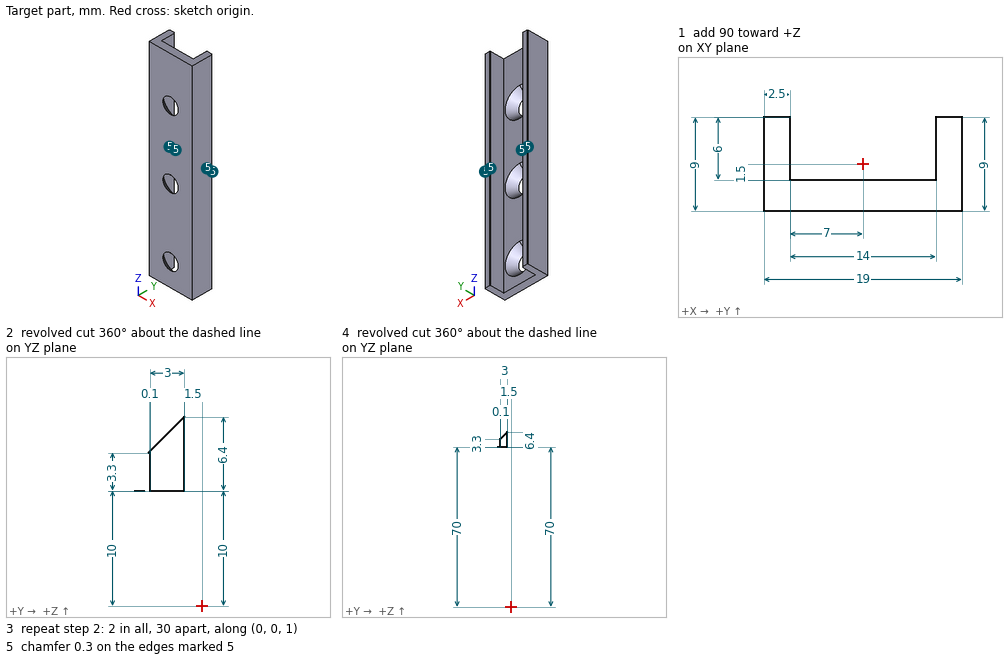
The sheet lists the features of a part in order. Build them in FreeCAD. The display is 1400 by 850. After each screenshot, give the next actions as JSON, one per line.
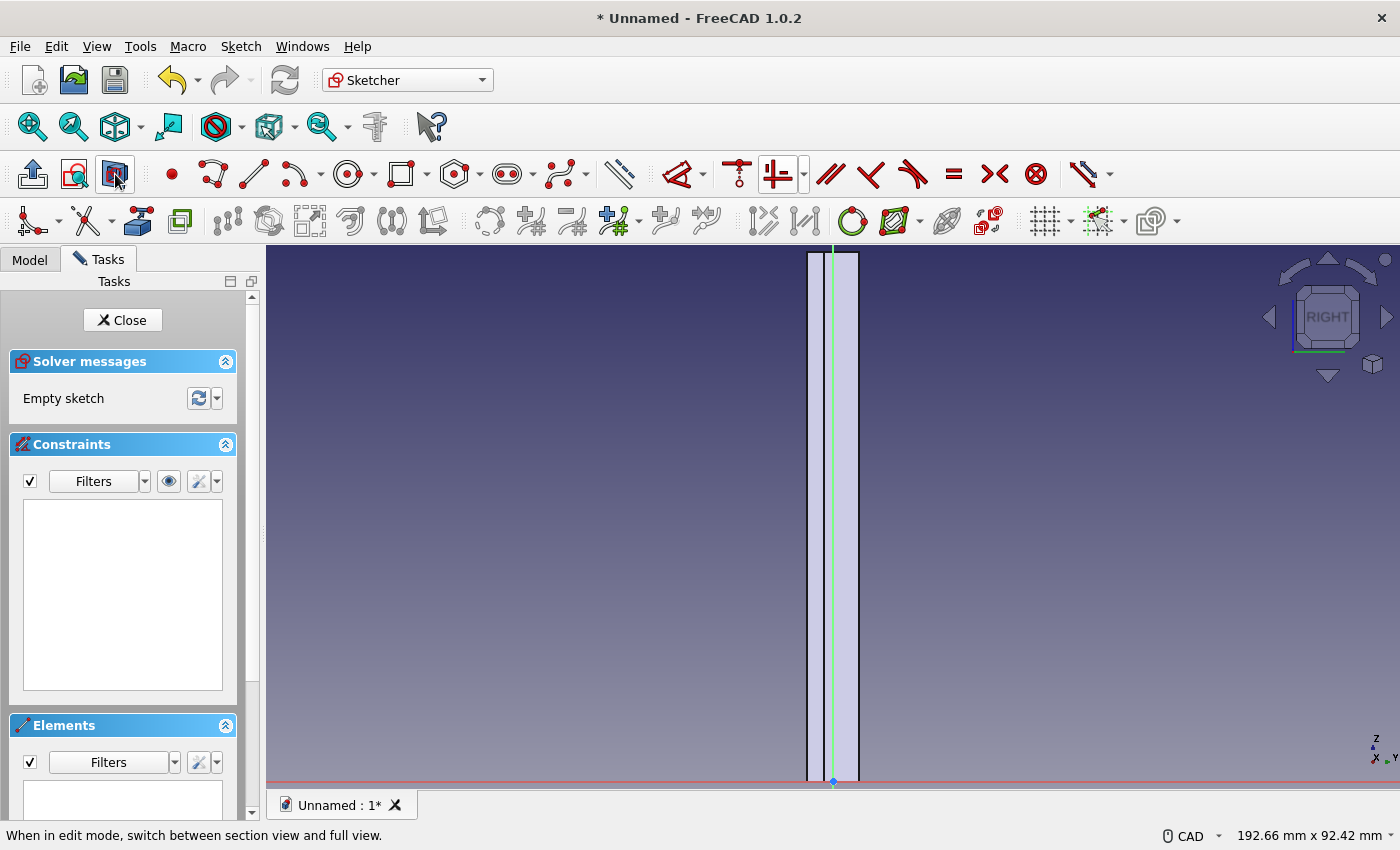
{"action": "scroll", "coordinate": [817, 727], "scroll_direction": "up", "scroll_amount": 11}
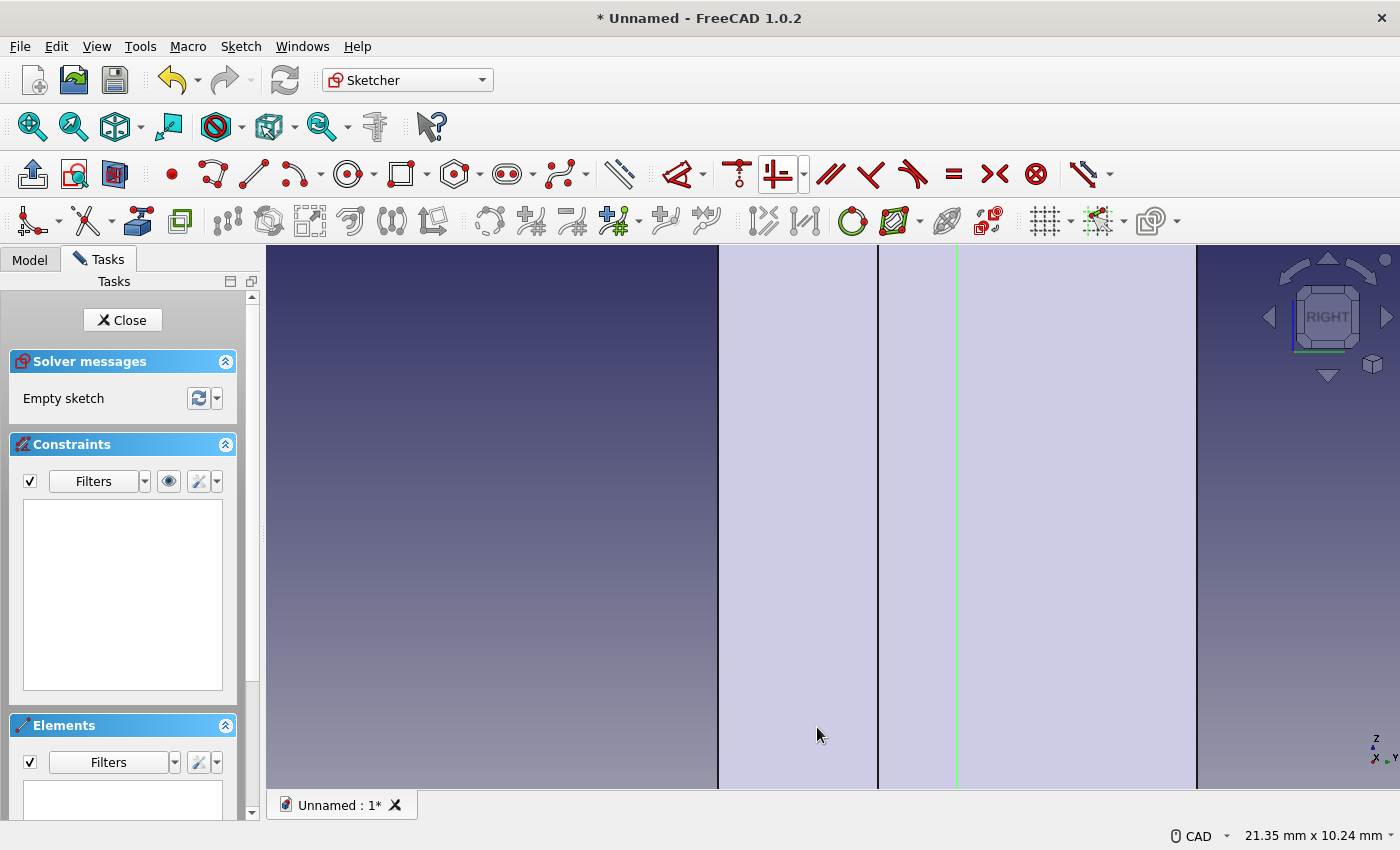
{"action": "left_click", "coordinate": [213, 174]}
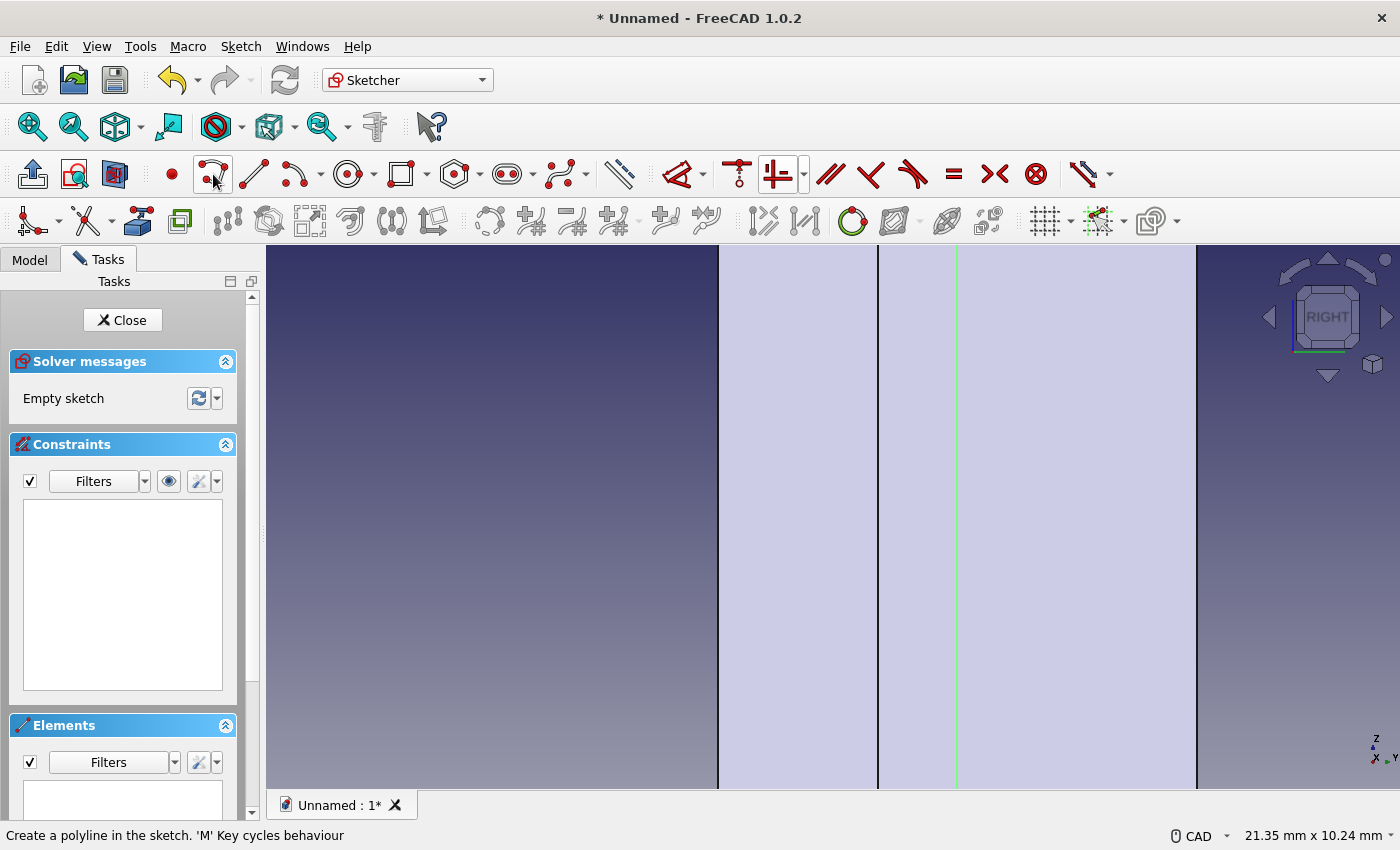
{"action": "left_click", "coordinate": [878, 684]}
{"action": "left_click", "coordinate": [878, 344]}
{"action": "left_click", "coordinate": [713, 509]}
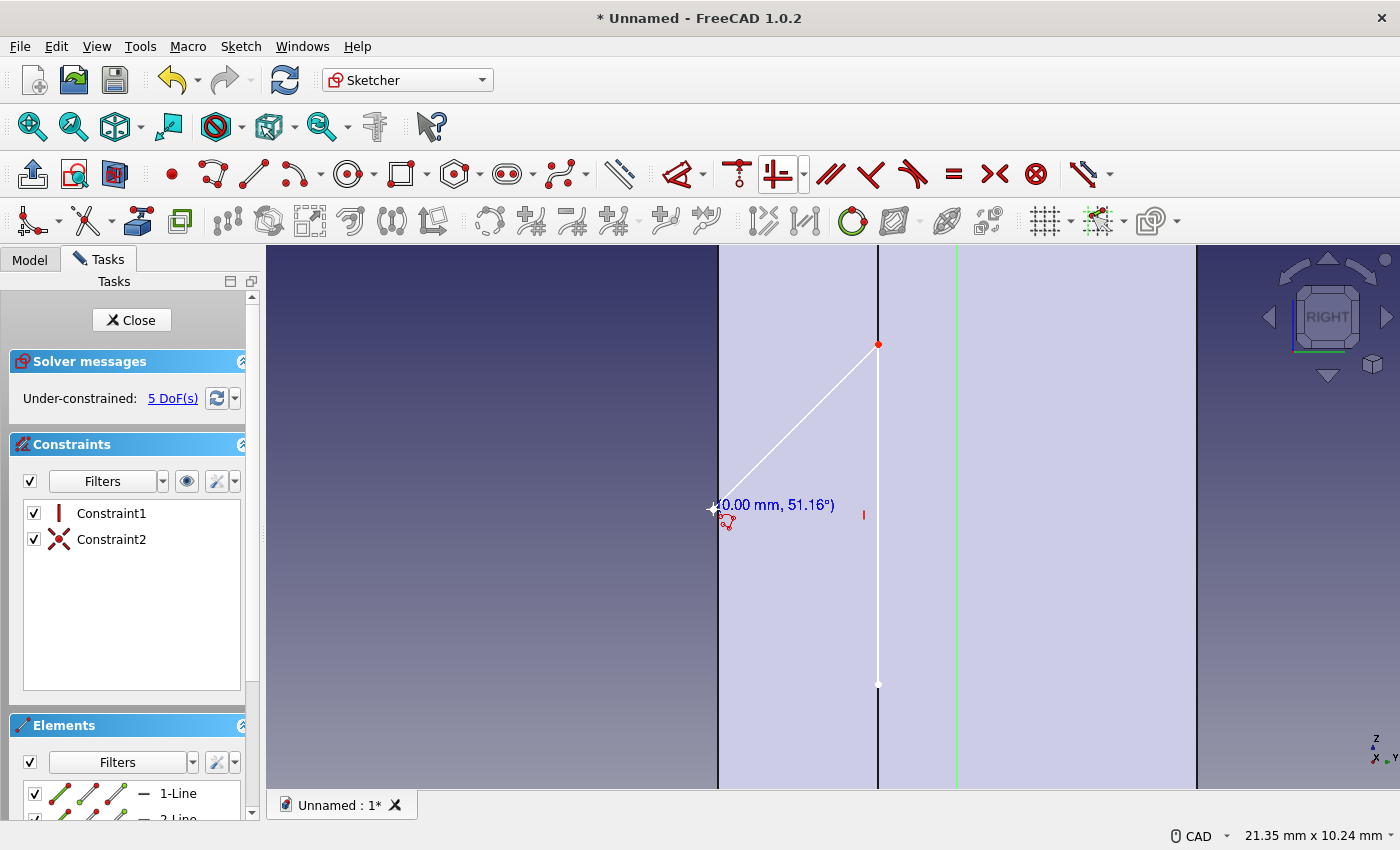
{"action": "scroll", "coordinate": [718, 509], "scroll_direction": "up", "scroll_amount": 8}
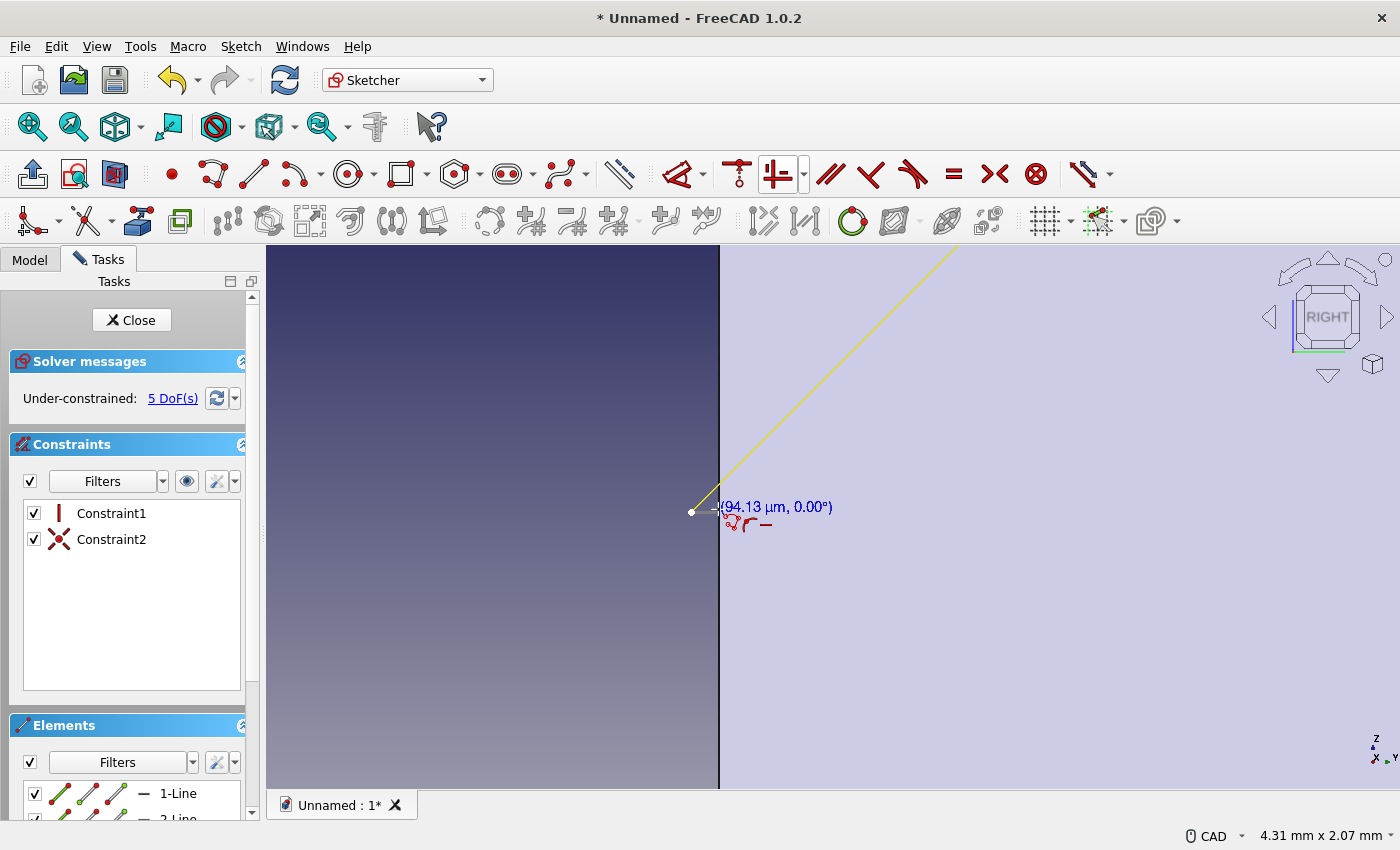
{"action": "left_click", "coordinate": [719, 507]}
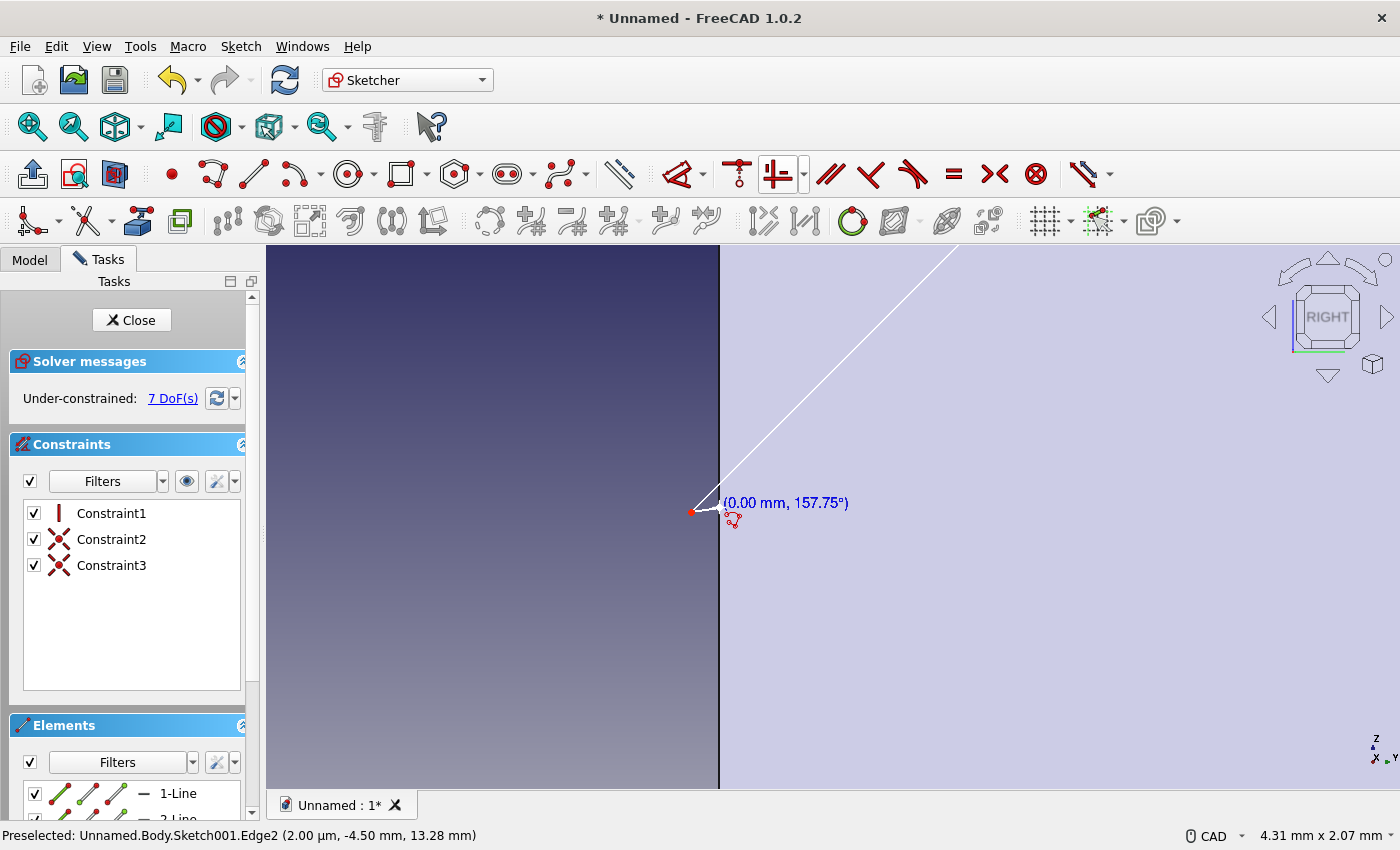
{"action": "scroll", "coordinate": [721, 513], "scroll_direction": "down", "scroll_amount": 8}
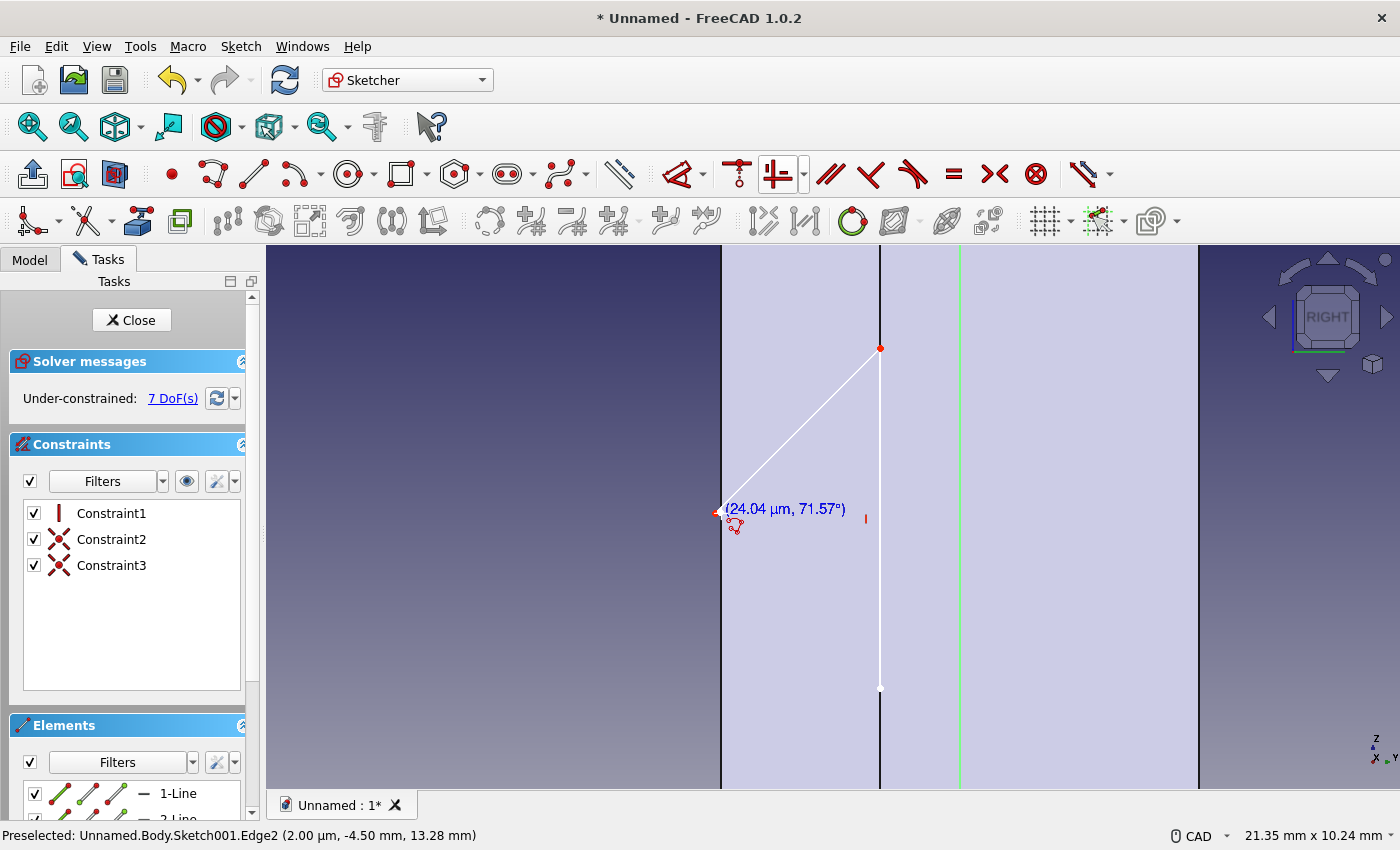
{"action": "left_click", "coordinate": [721, 687]}
{"action": "left_click", "coordinate": [880, 688]}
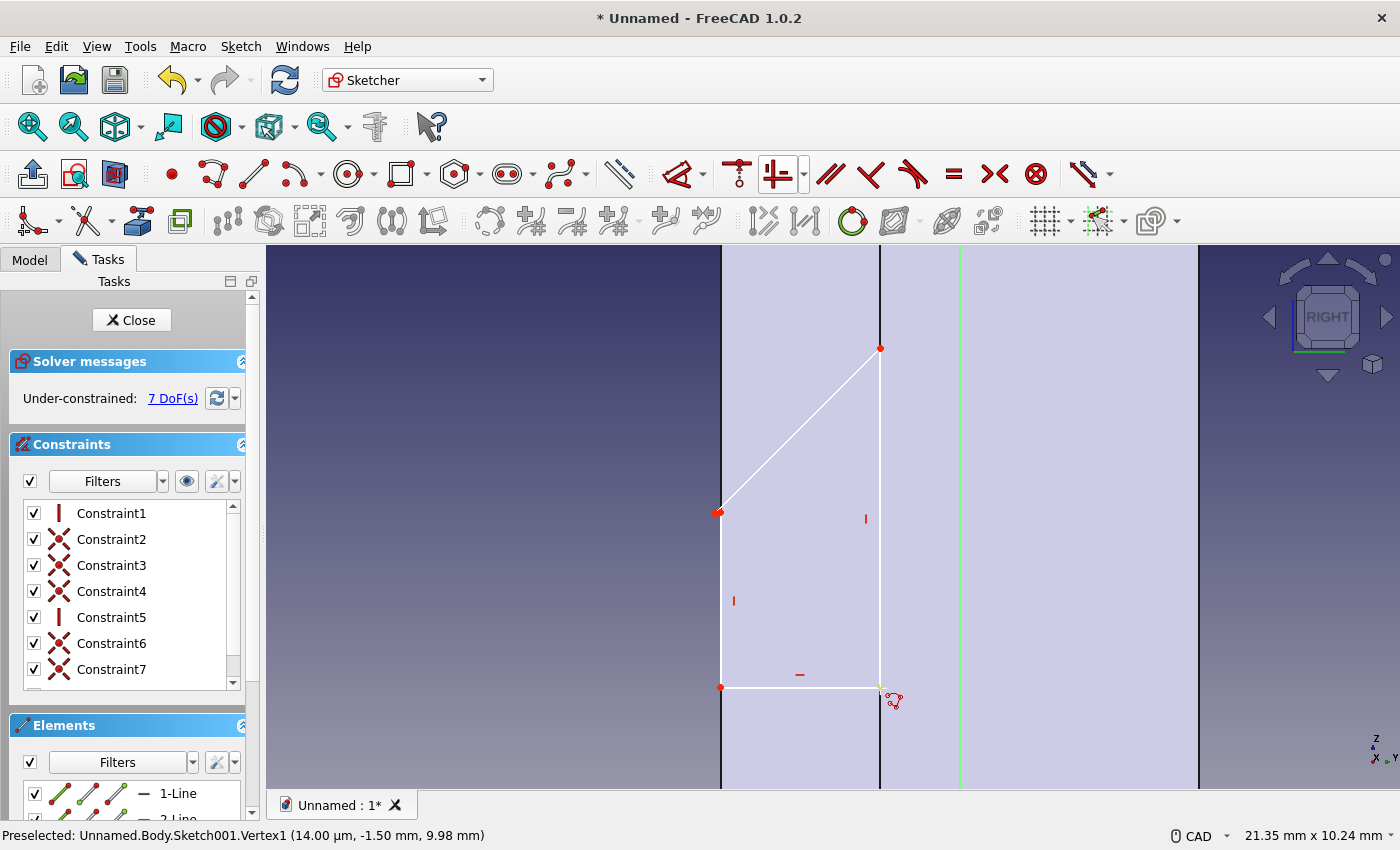
{"action": "left_click", "coordinate": [254, 174]}